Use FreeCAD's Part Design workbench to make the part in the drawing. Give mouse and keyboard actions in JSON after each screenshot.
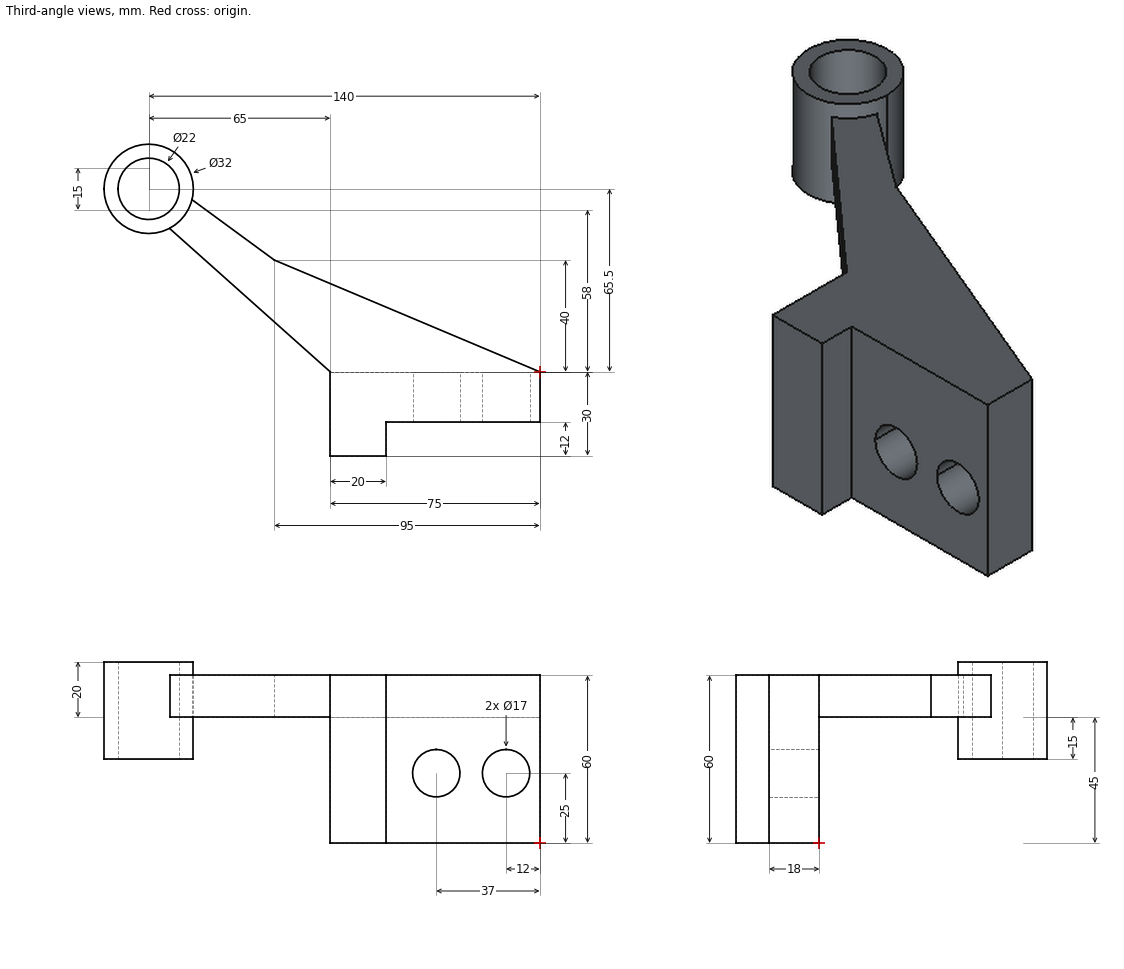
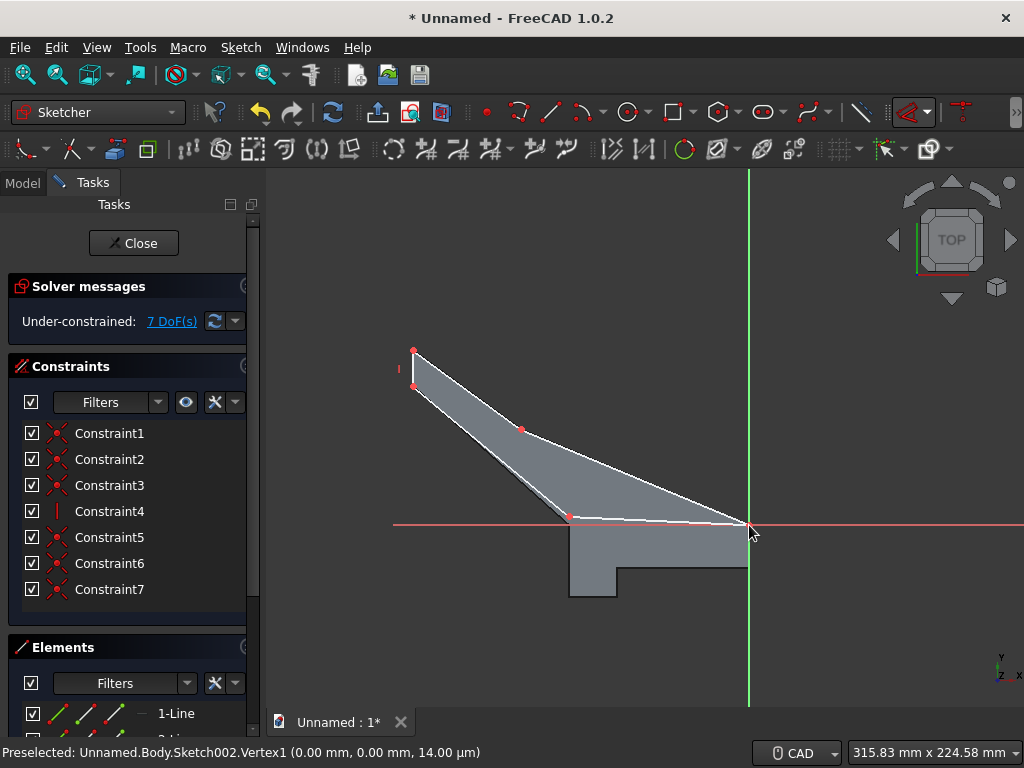
{"action": "left_click", "coordinate": [695, 523]}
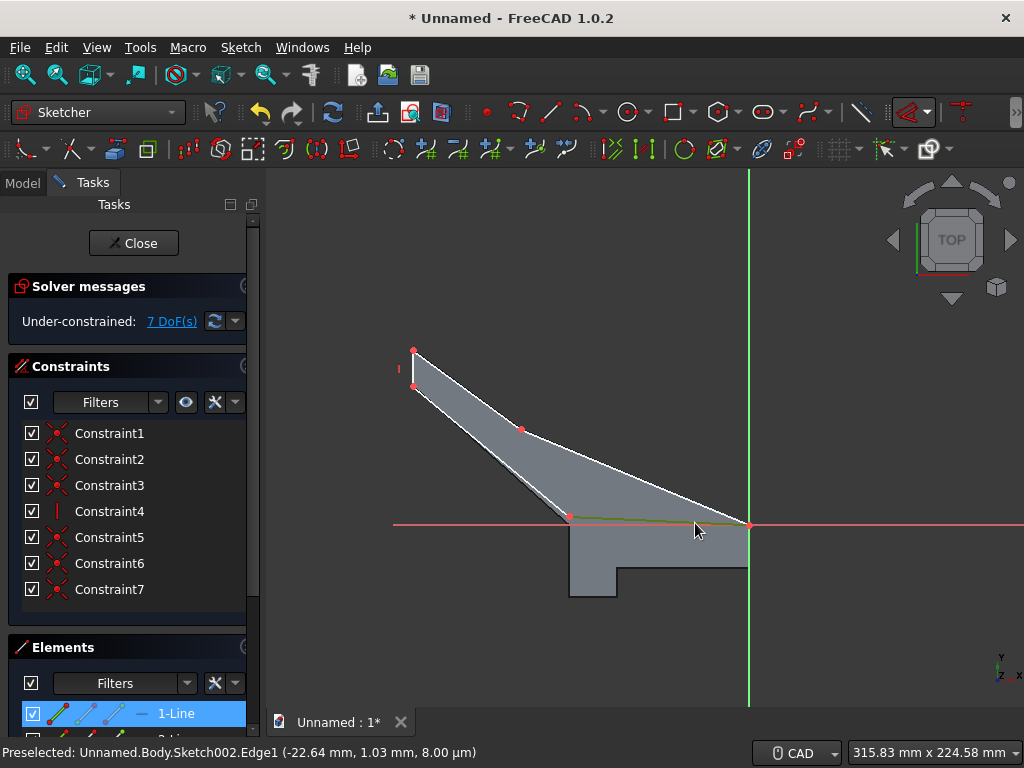
{"action": "key", "text": "h"}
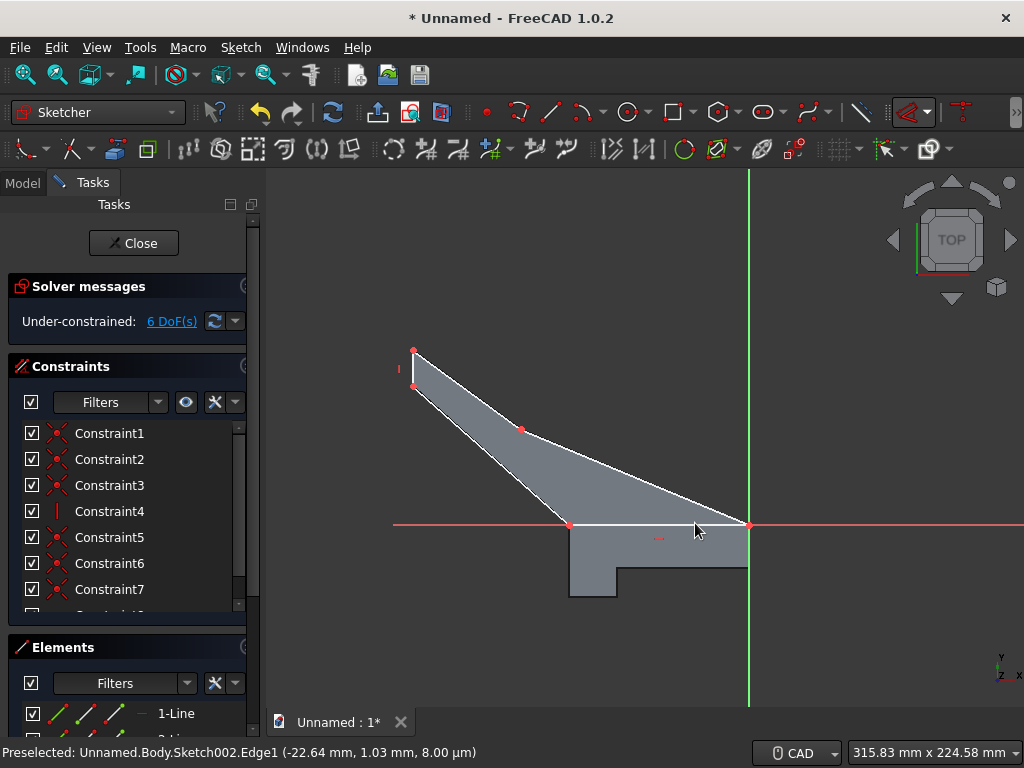
{"action": "left_click", "coordinate": [695, 525]}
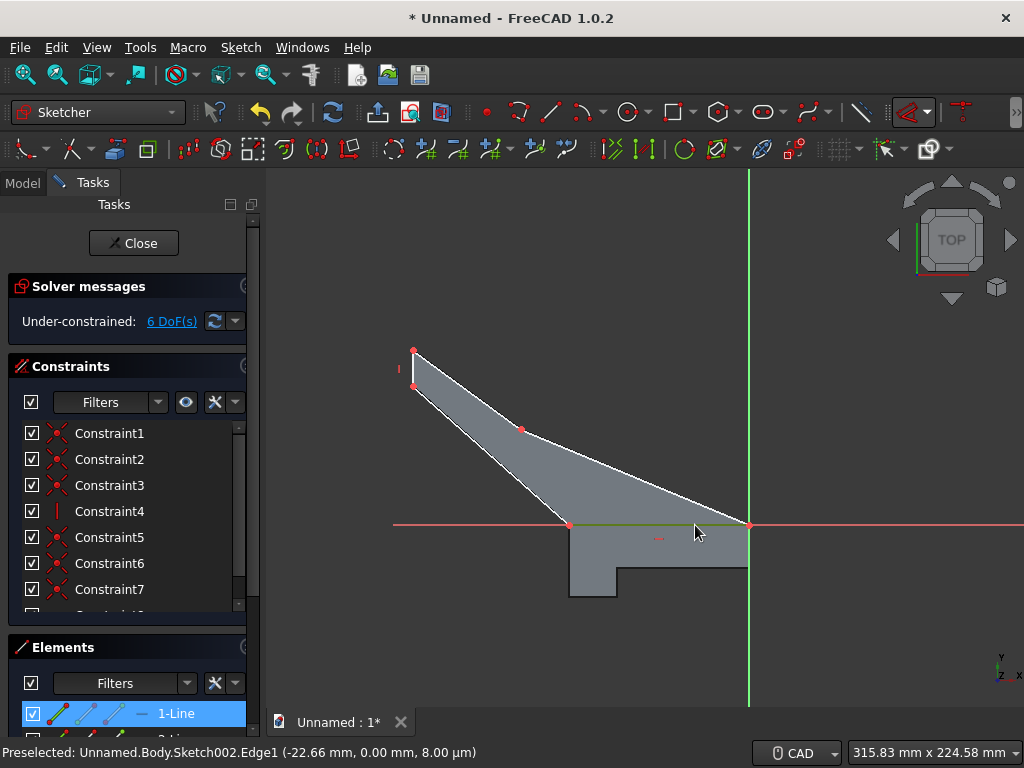
{"action": "left_click", "coordinate": [930, 112]}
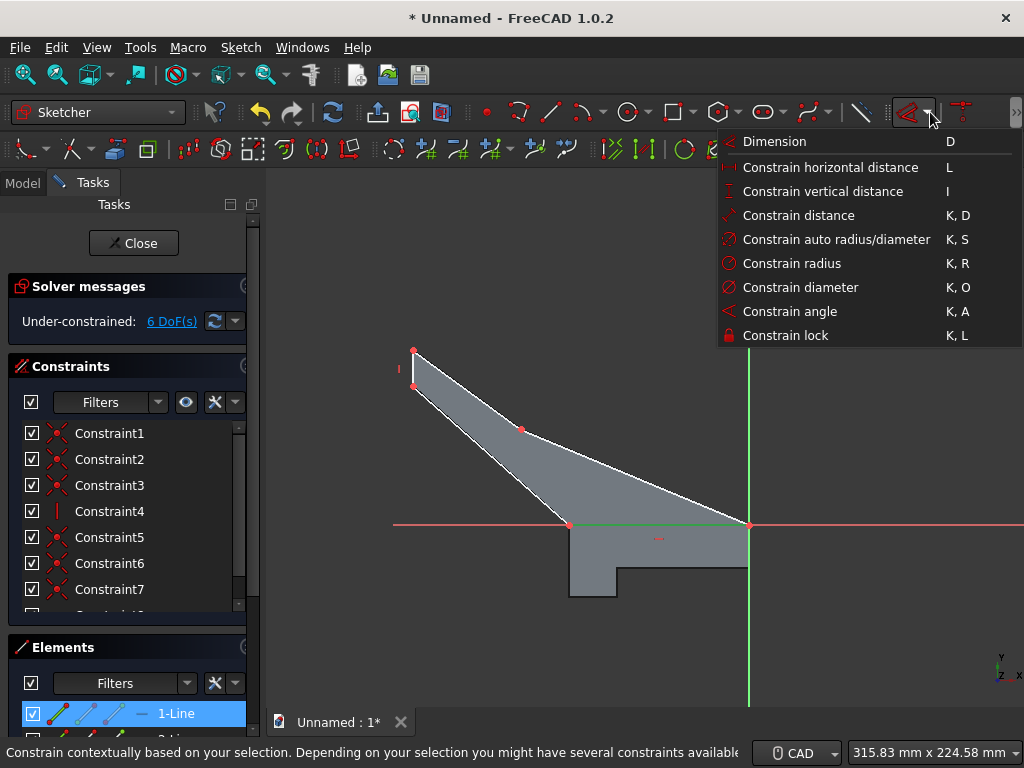
{"action": "left_click", "coordinate": [870, 167]}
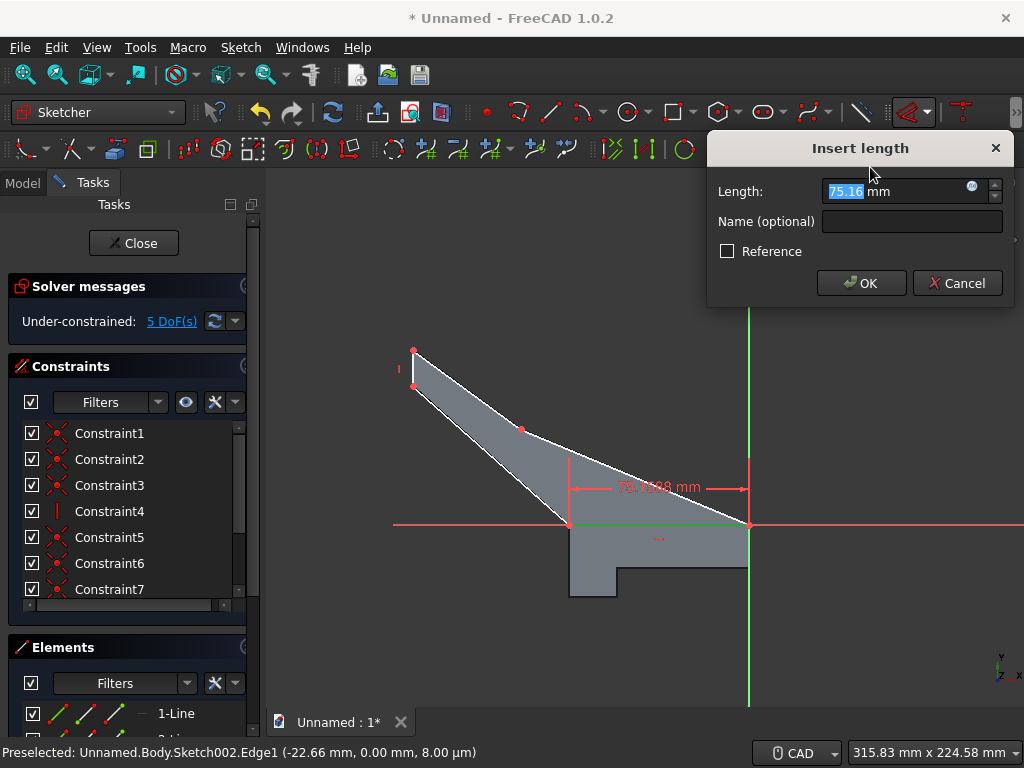
{"action": "type", "text": "75"}
{"action": "key", "text": "Return"}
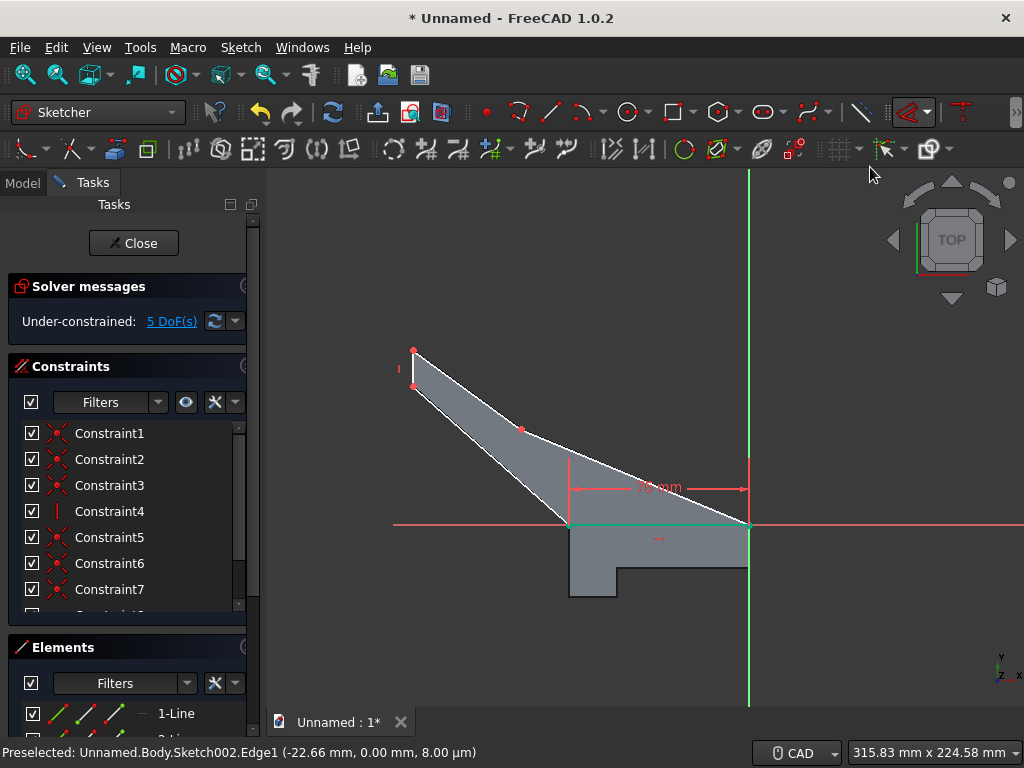
{"action": "scroll", "coordinate": [413, 376], "scroll_direction": "up", "scroll_amount": 2}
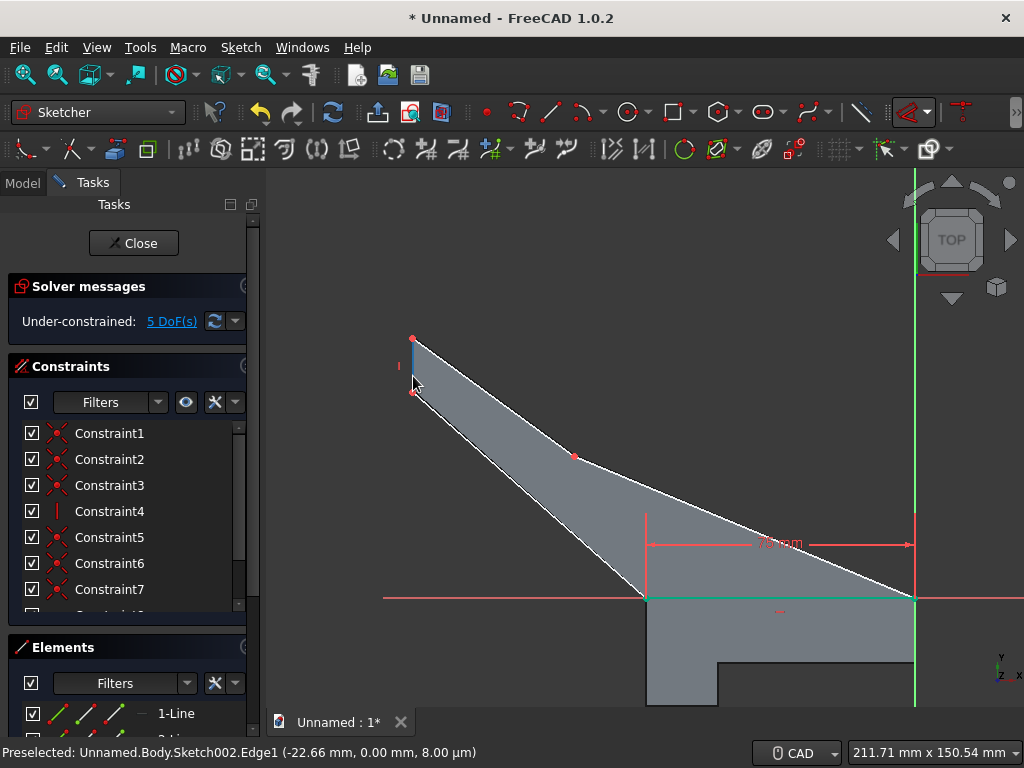
{"action": "left_click", "coordinate": [413, 376]}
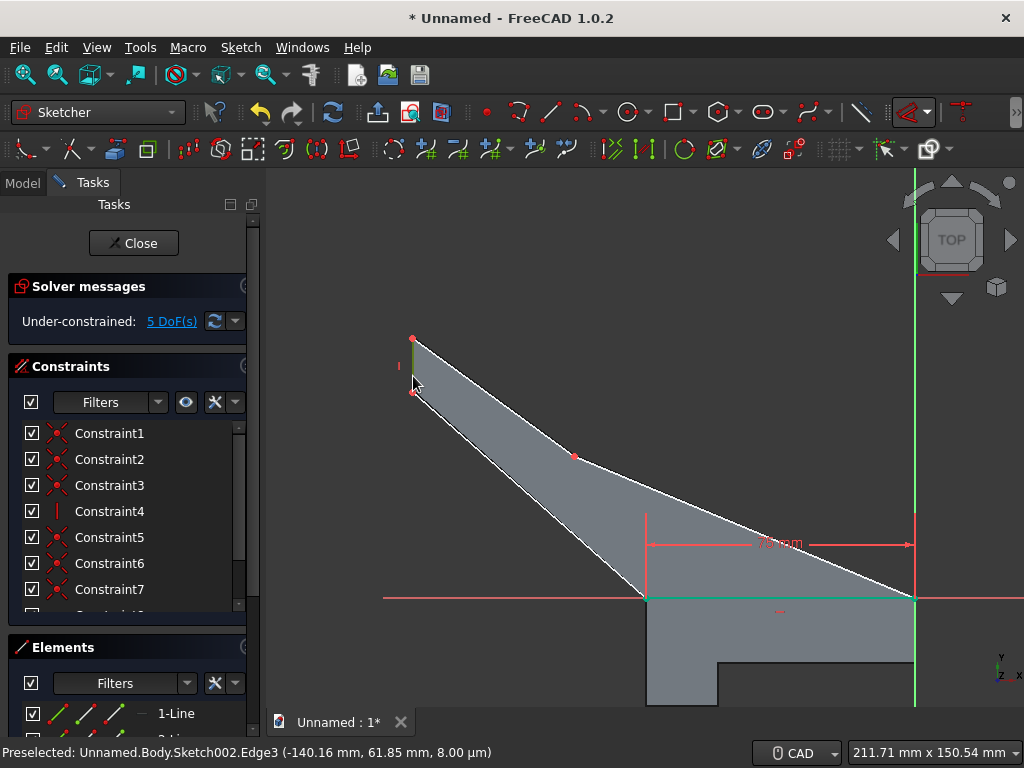
{"action": "left_click", "coordinate": [930, 112]}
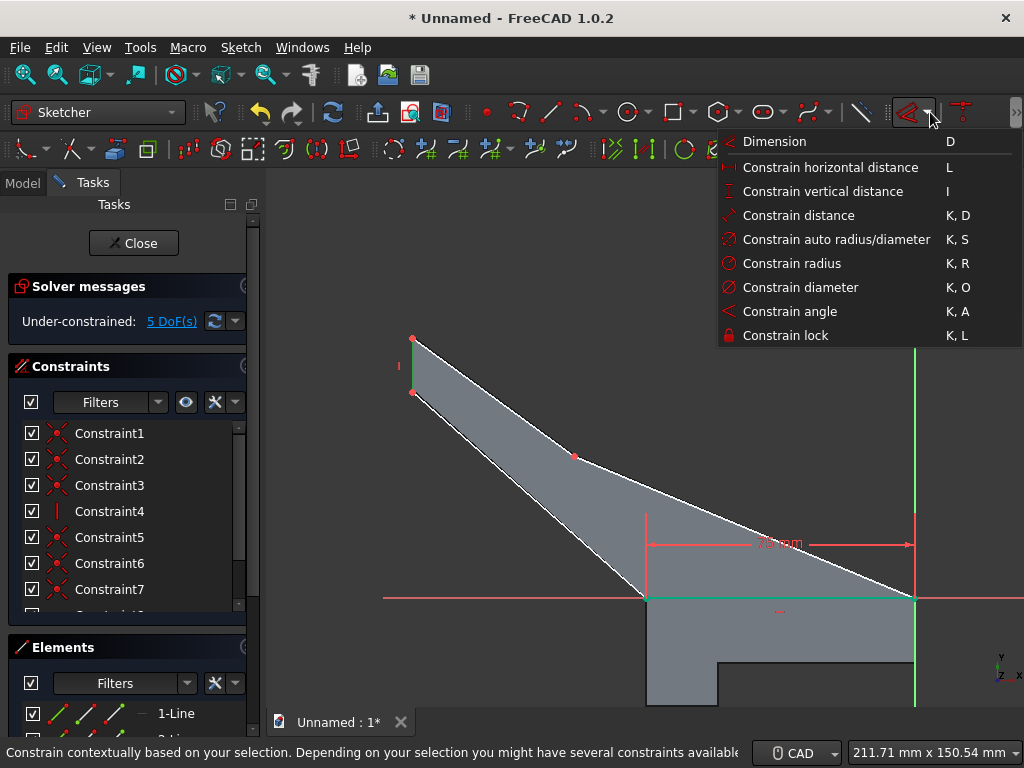
{"action": "left_click", "coordinate": [870, 191]}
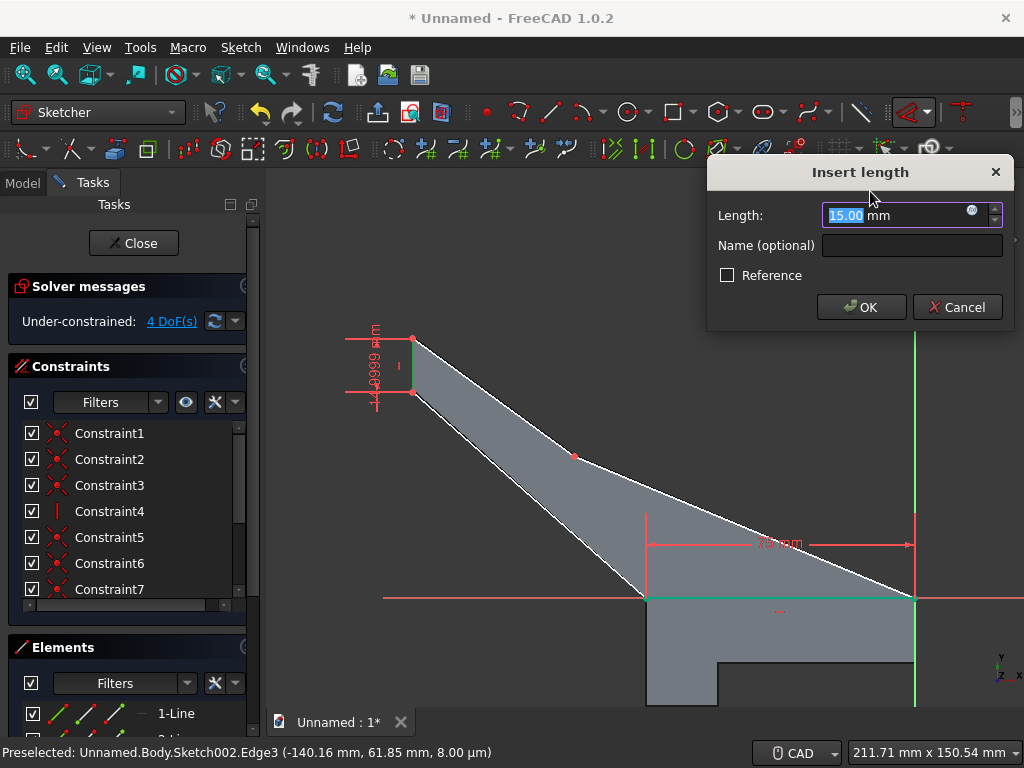
{"action": "type", "text": "15"}
{"action": "key", "text": "Return"}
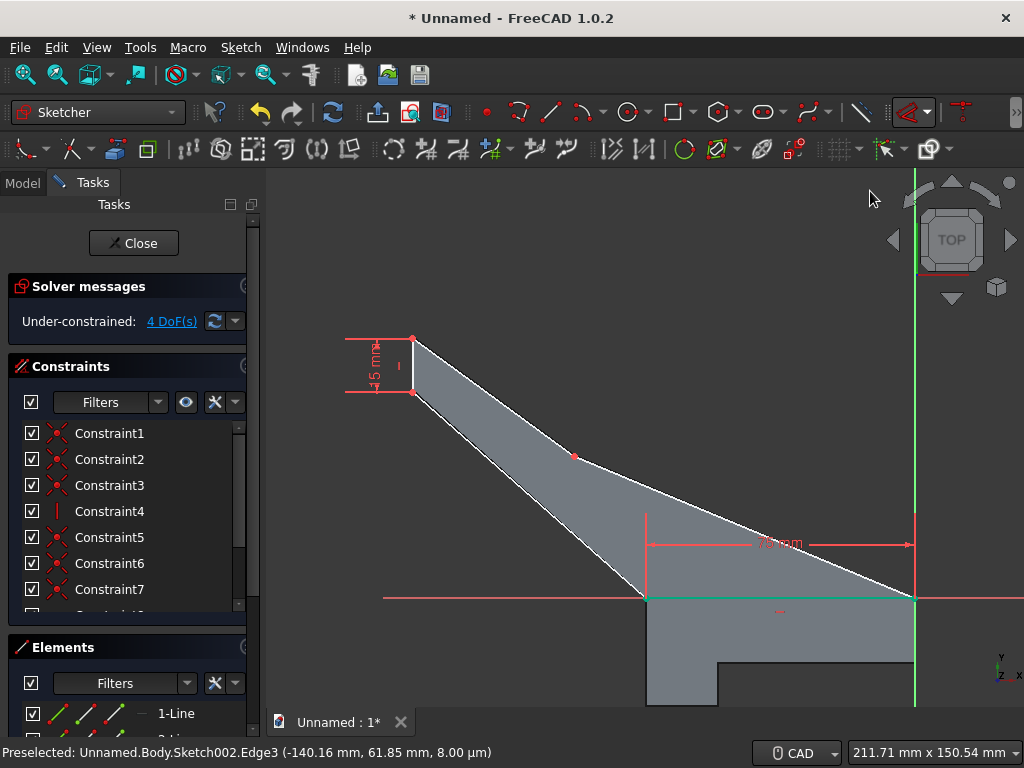
{"action": "left_click", "coordinate": [413, 392]}